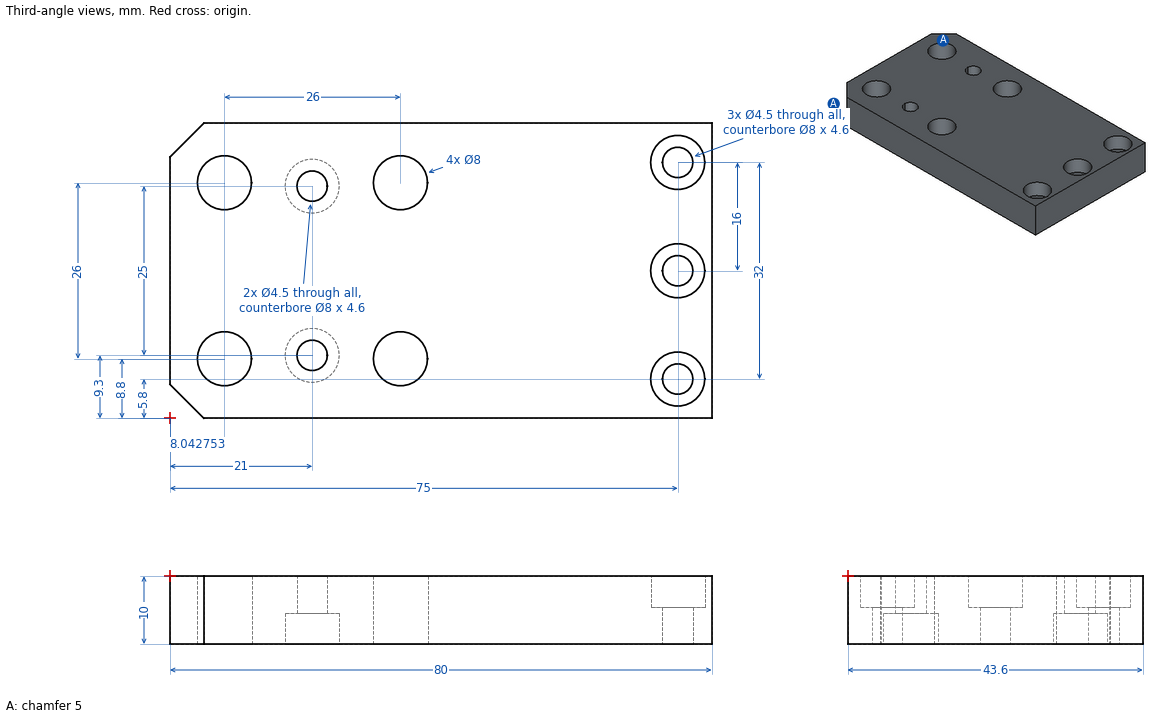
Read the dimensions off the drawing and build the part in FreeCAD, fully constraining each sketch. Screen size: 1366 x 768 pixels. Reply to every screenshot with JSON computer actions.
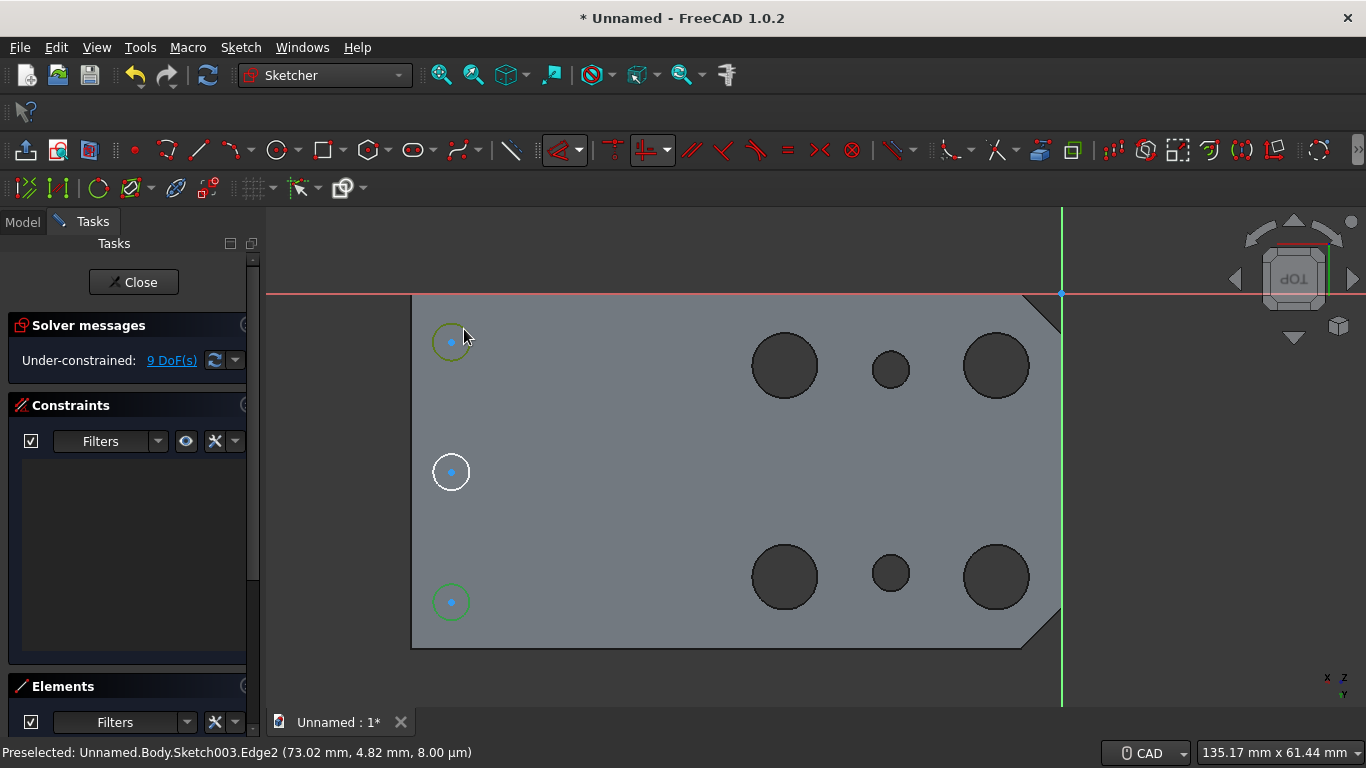
{"action": "left_click", "coordinate": [464, 459]}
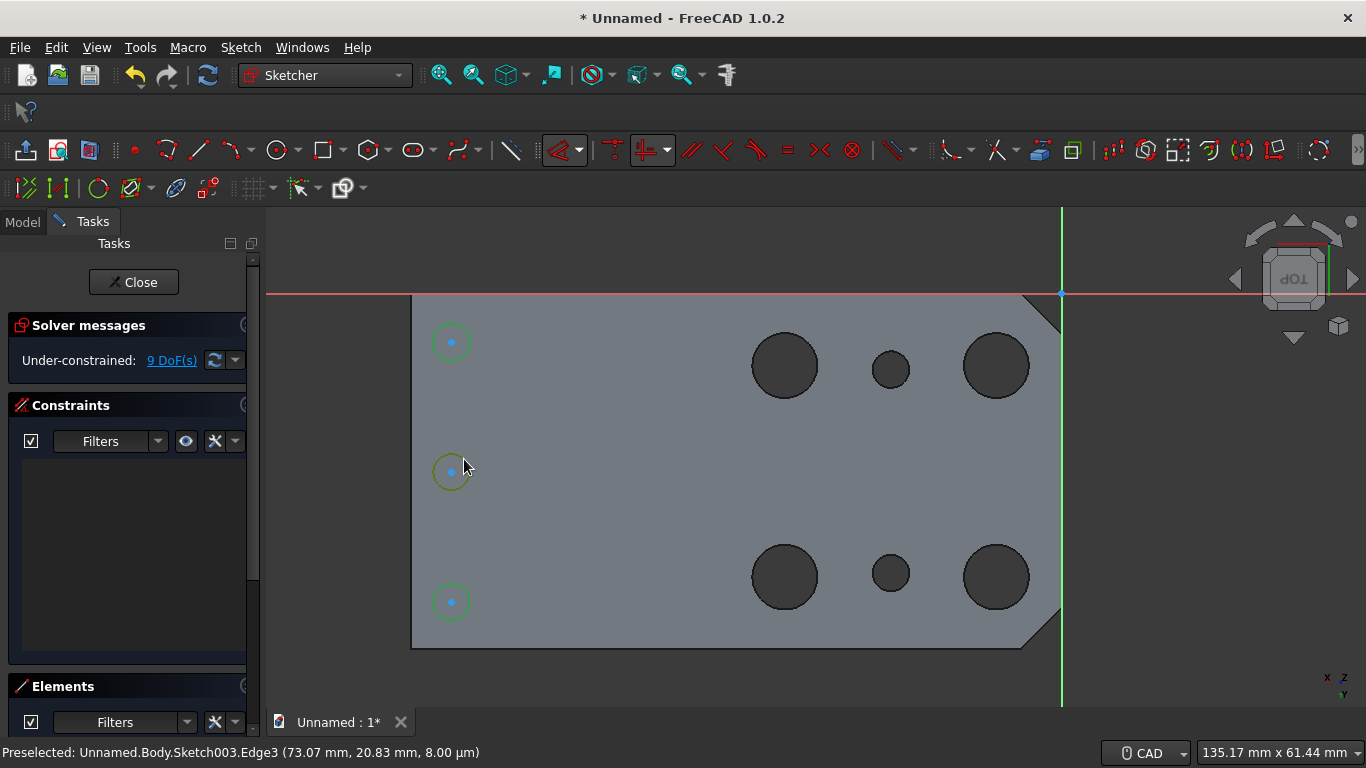
{"action": "left_click", "coordinate": [788, 150]}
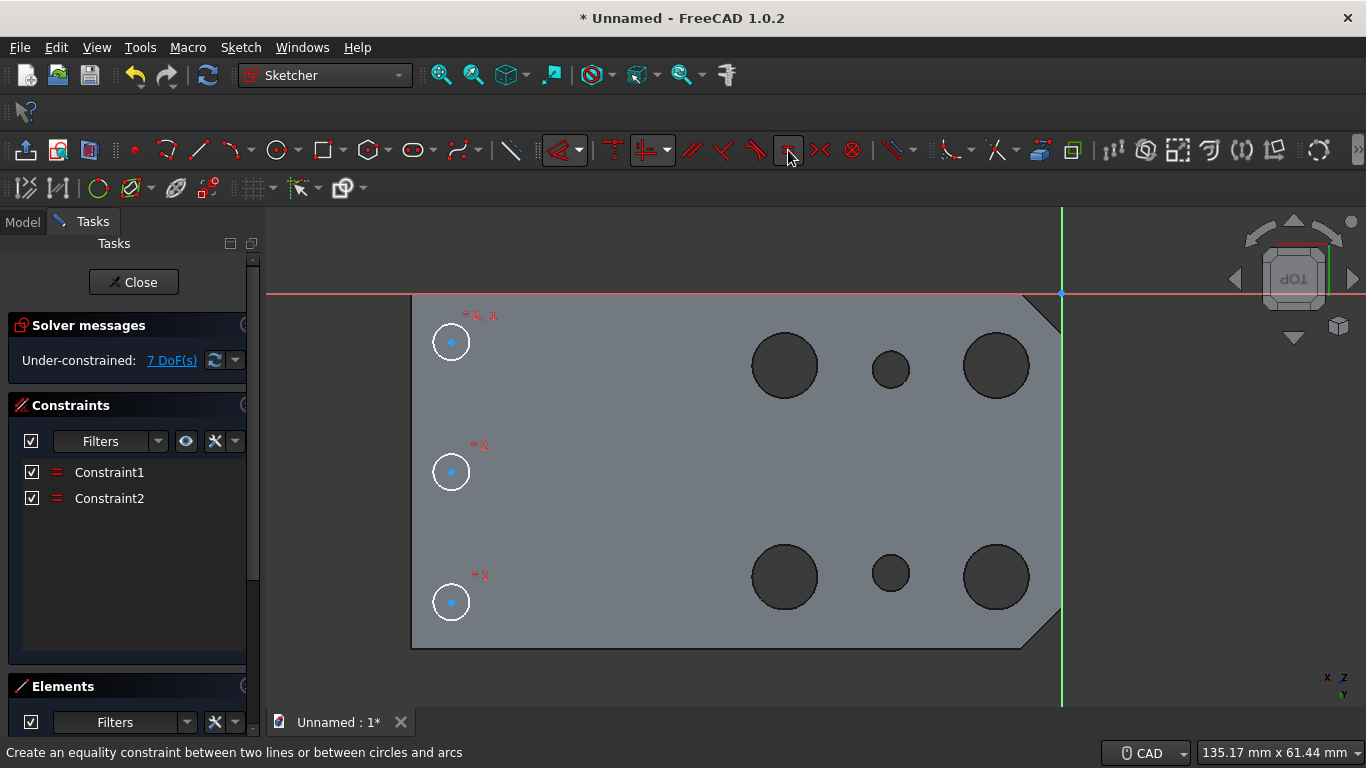
{"action": "left_click", "coordinate": [464, 589]}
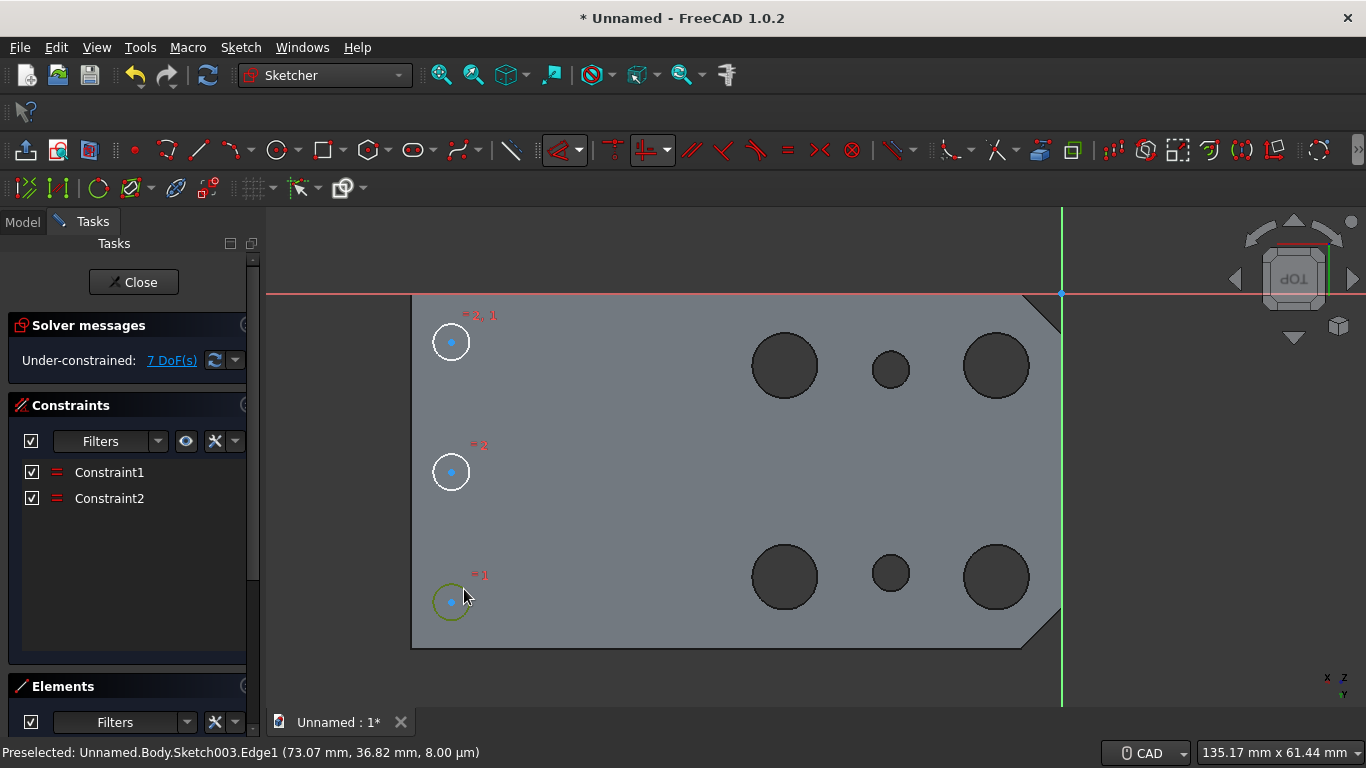
{"action": "left_click", "coordinate": [582, 150]}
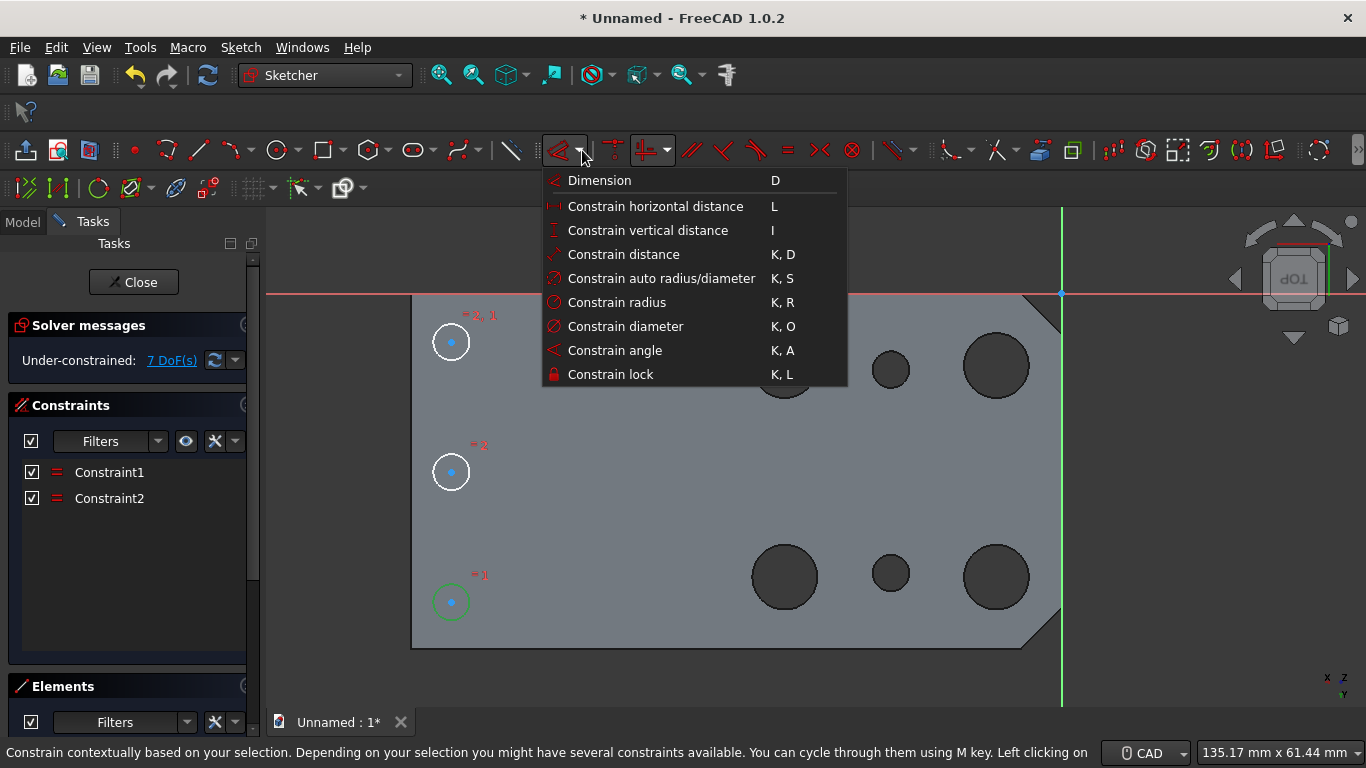
{"action": "left_click", "coordinate": [695, 326]}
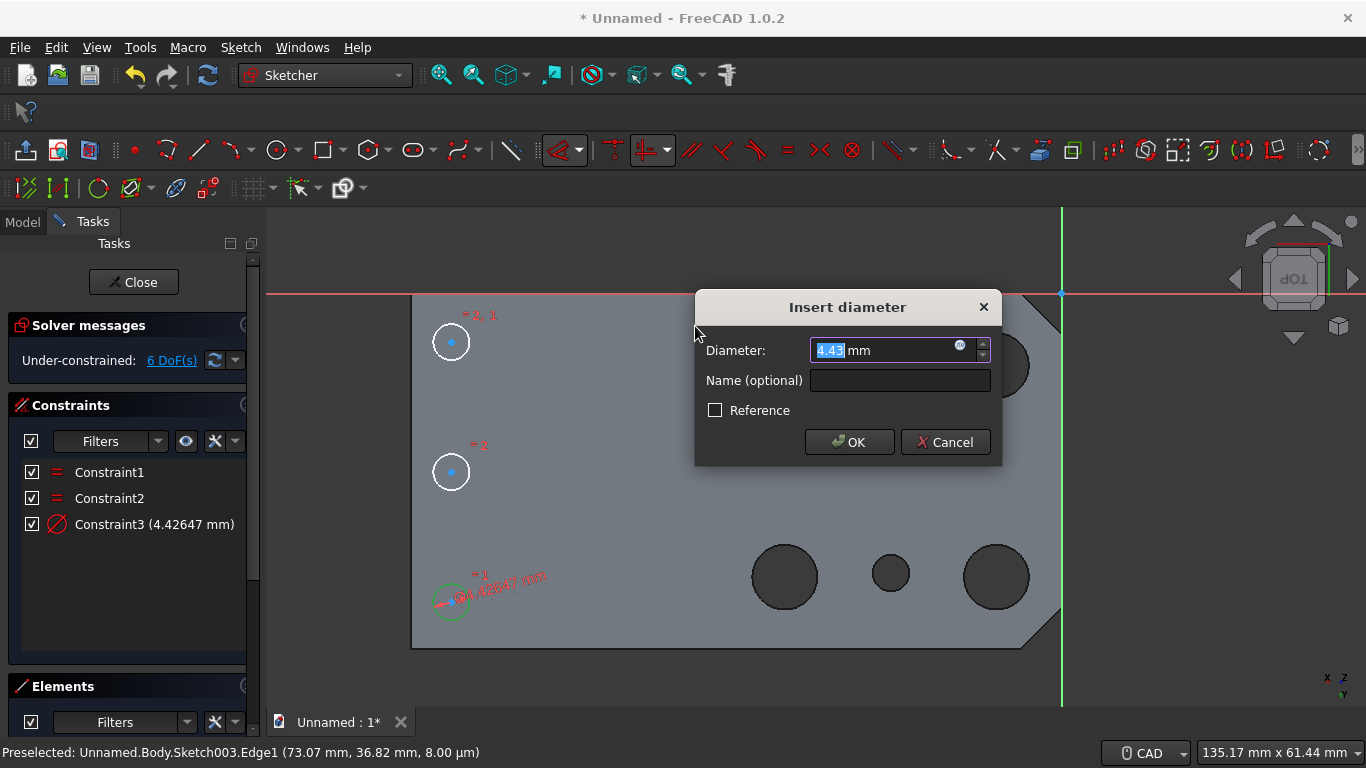
{"action": "type", "text": "4.5"}
{"action": "key", "text": "Return"}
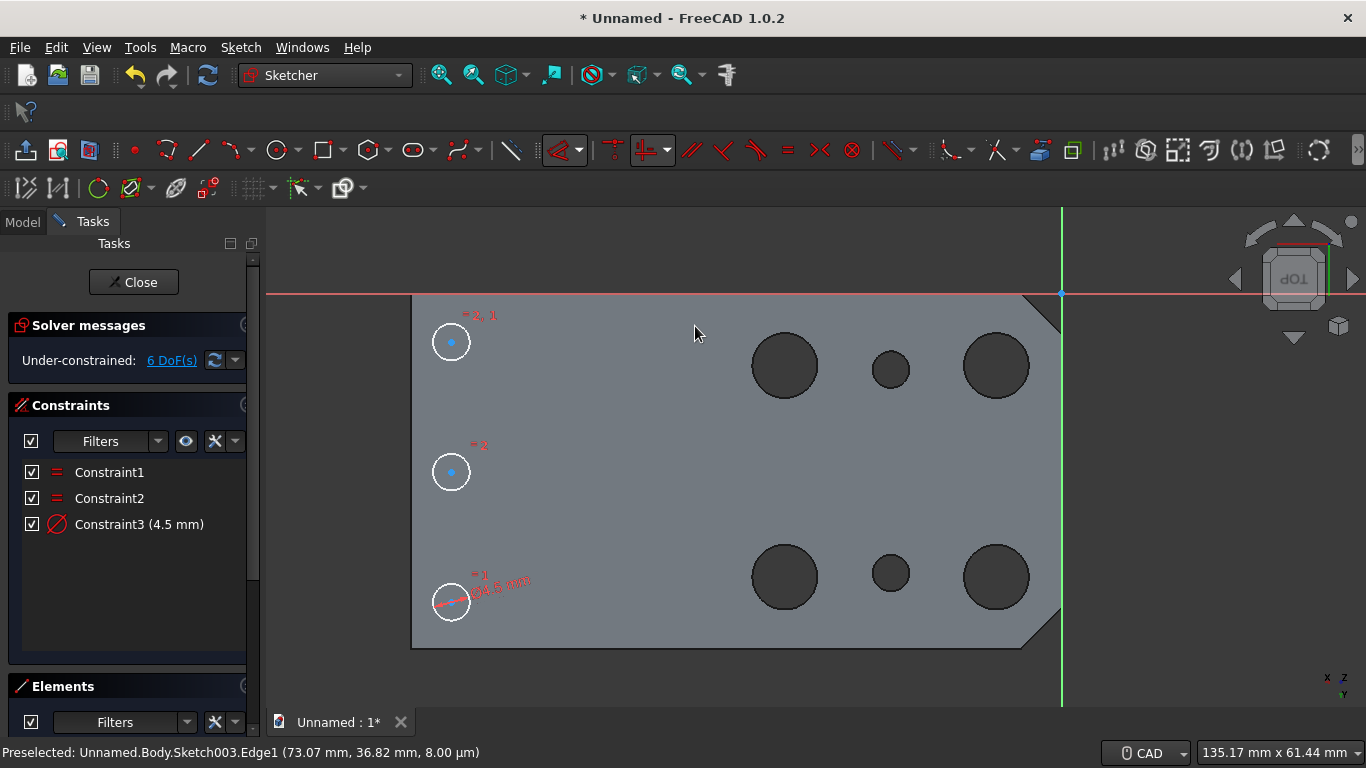
{"action": "left_click", "coordinate": [451, 602]}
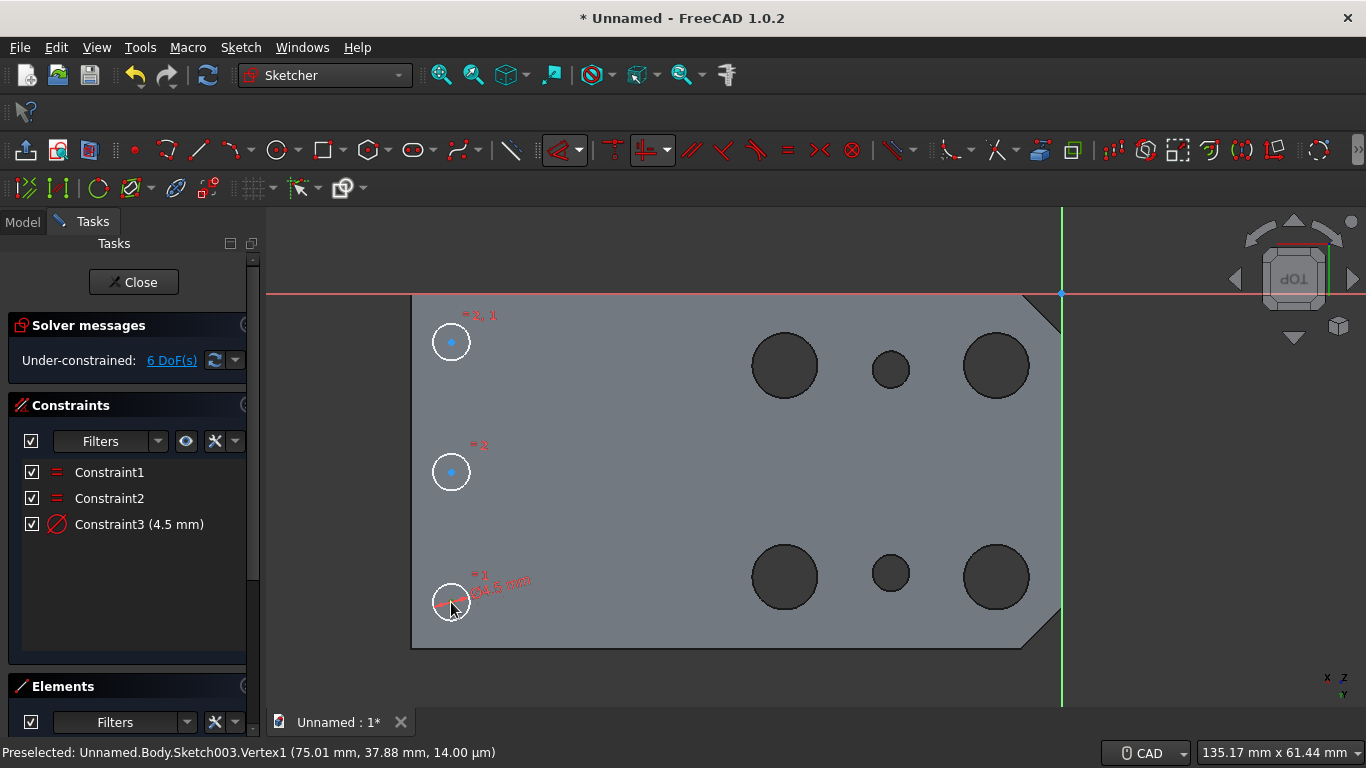
{"action": "left_click", "coordinate": [582, 150]}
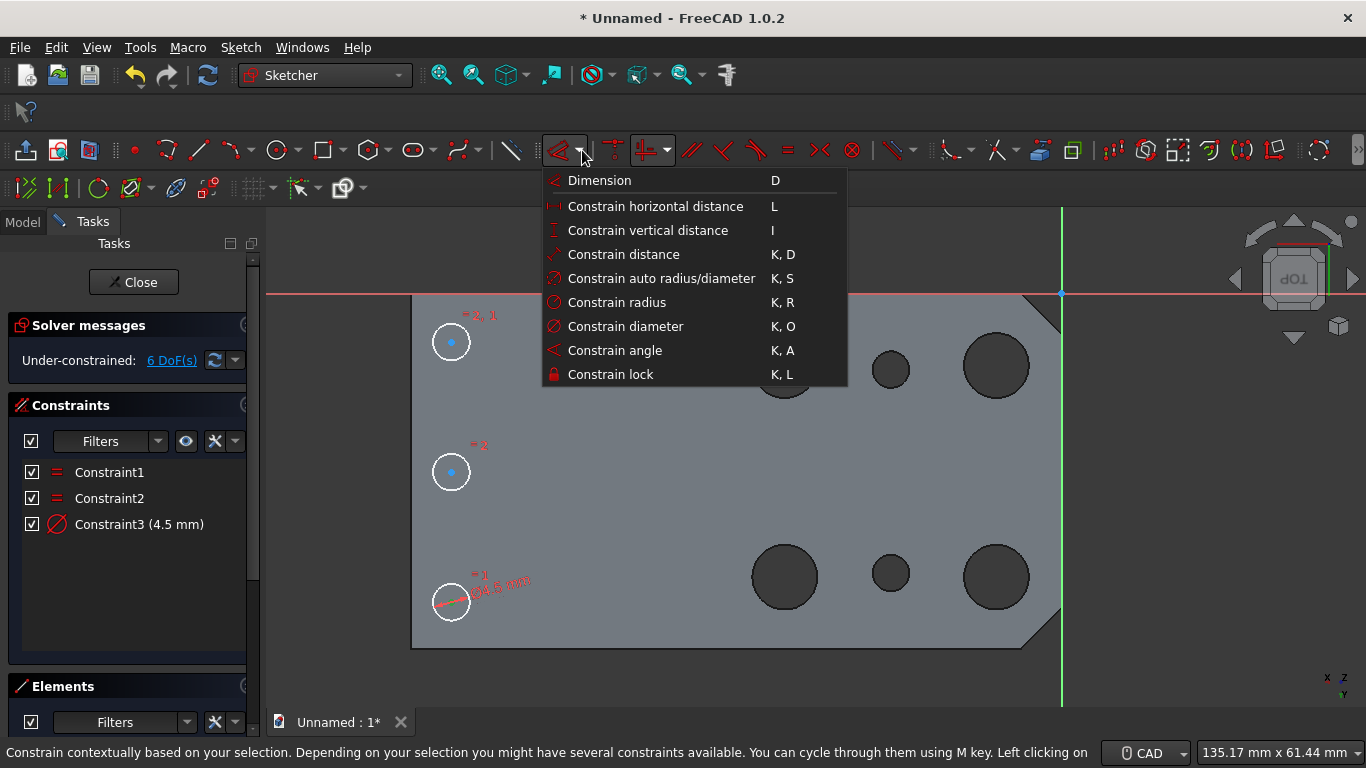
{"action": "left_click", "coordinate": [695, 206]}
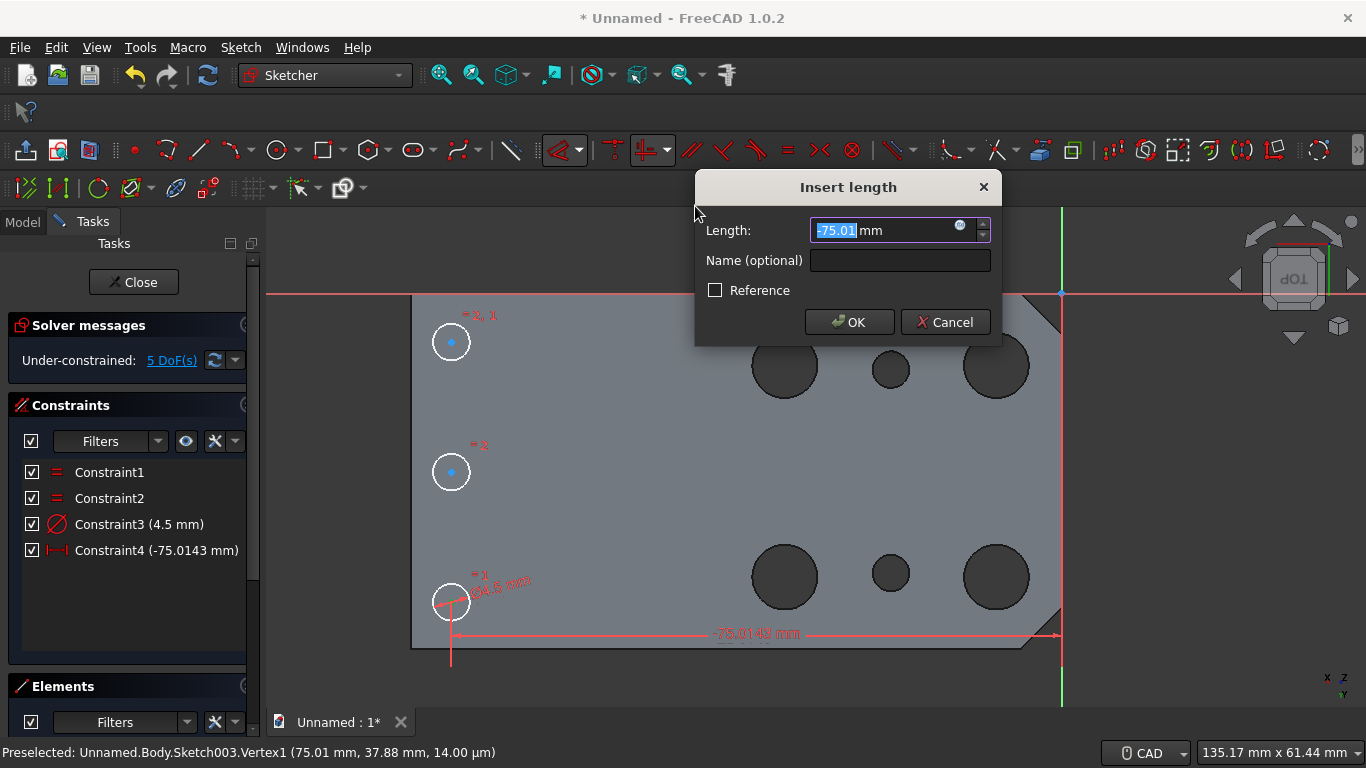
{"action": "type", "text": "-75"}
{"action": "key", "text": "Return"}